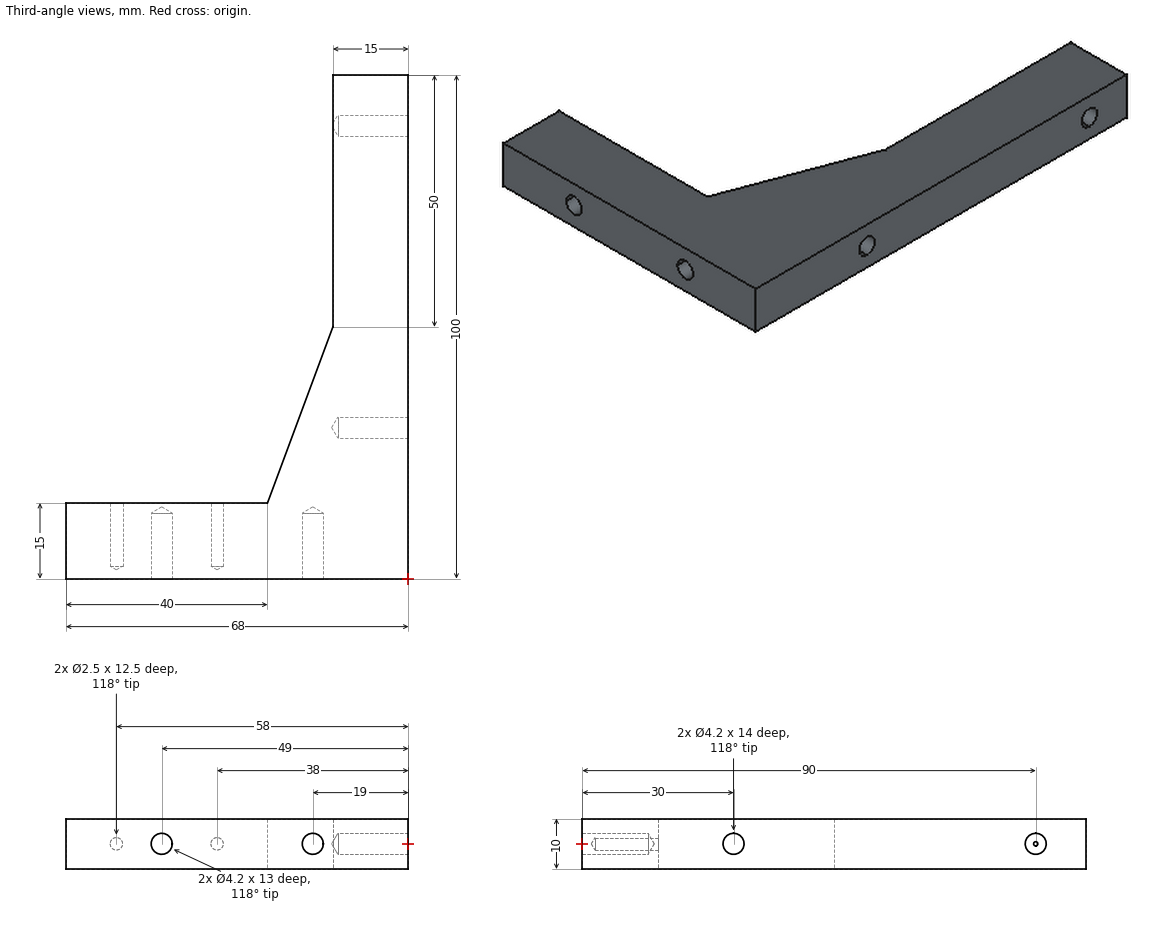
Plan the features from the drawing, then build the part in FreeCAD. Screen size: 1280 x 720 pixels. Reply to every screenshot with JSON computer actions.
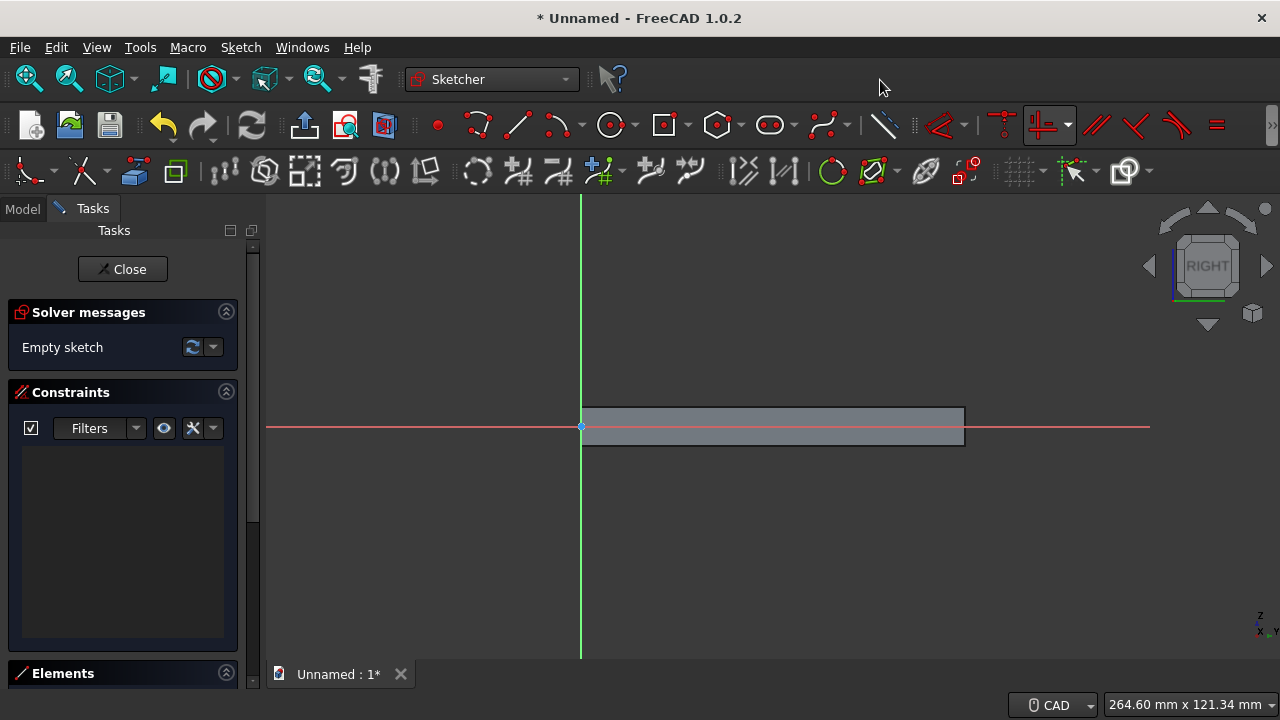
{"action": "scroll", "coordinate": [866, 426], "scroll_direction": "up", "scroll_amount": 2}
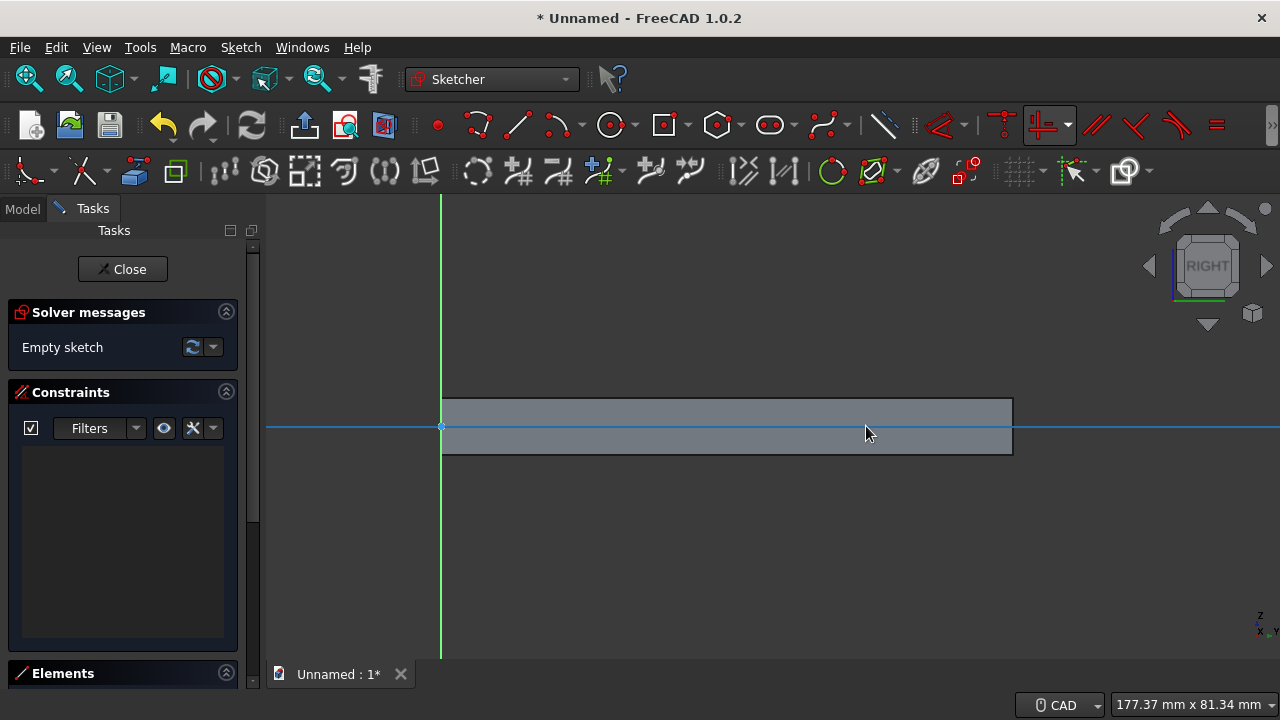
{"action": "key", "text": "g c"}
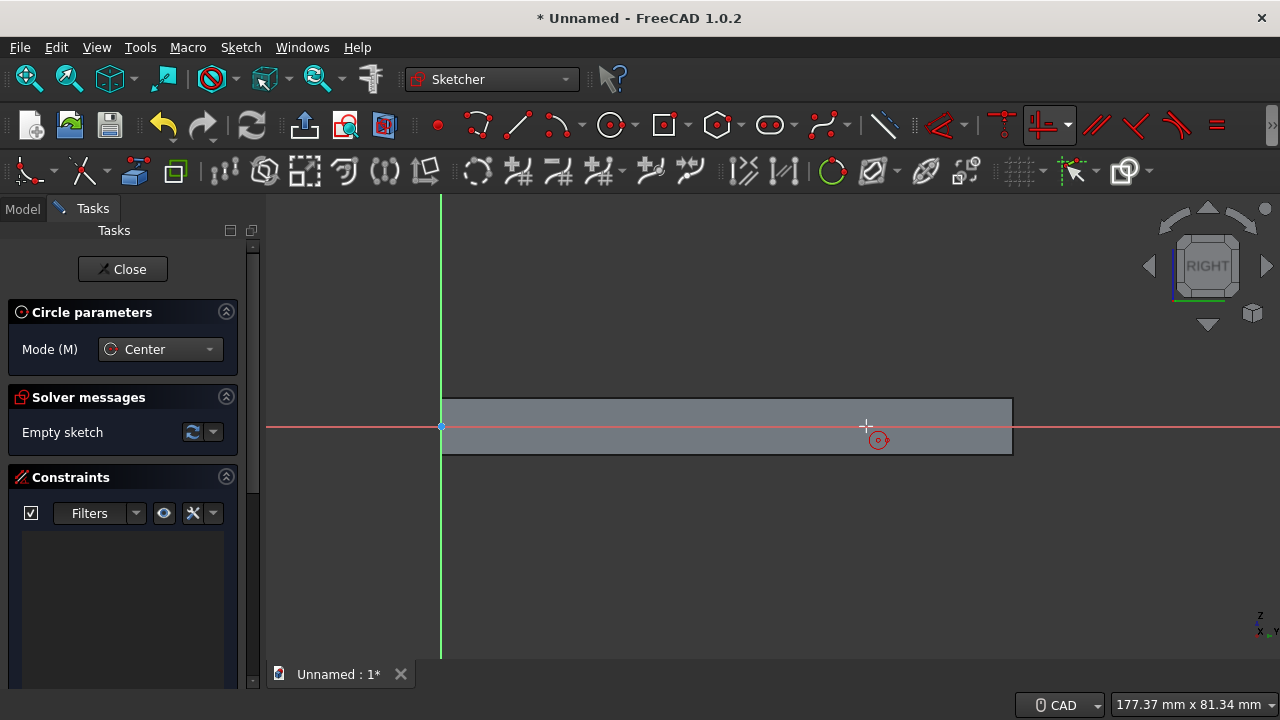
{"action": "scroll", "coordinate": [613, 426], "scroll_direction": "up", "scroll_amount": 4}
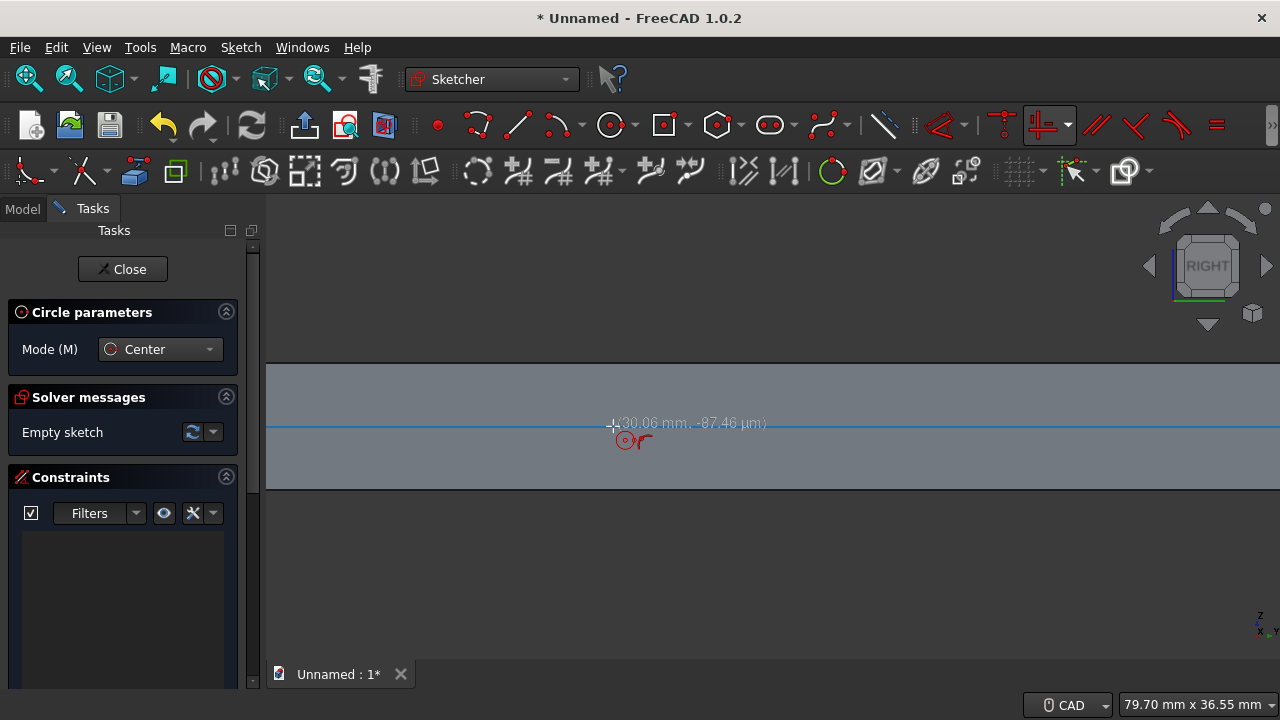
{"action": "left_click", "coordinate": [612, 426]}
{"action": "mouse_move", "coordinate": [631, 408]}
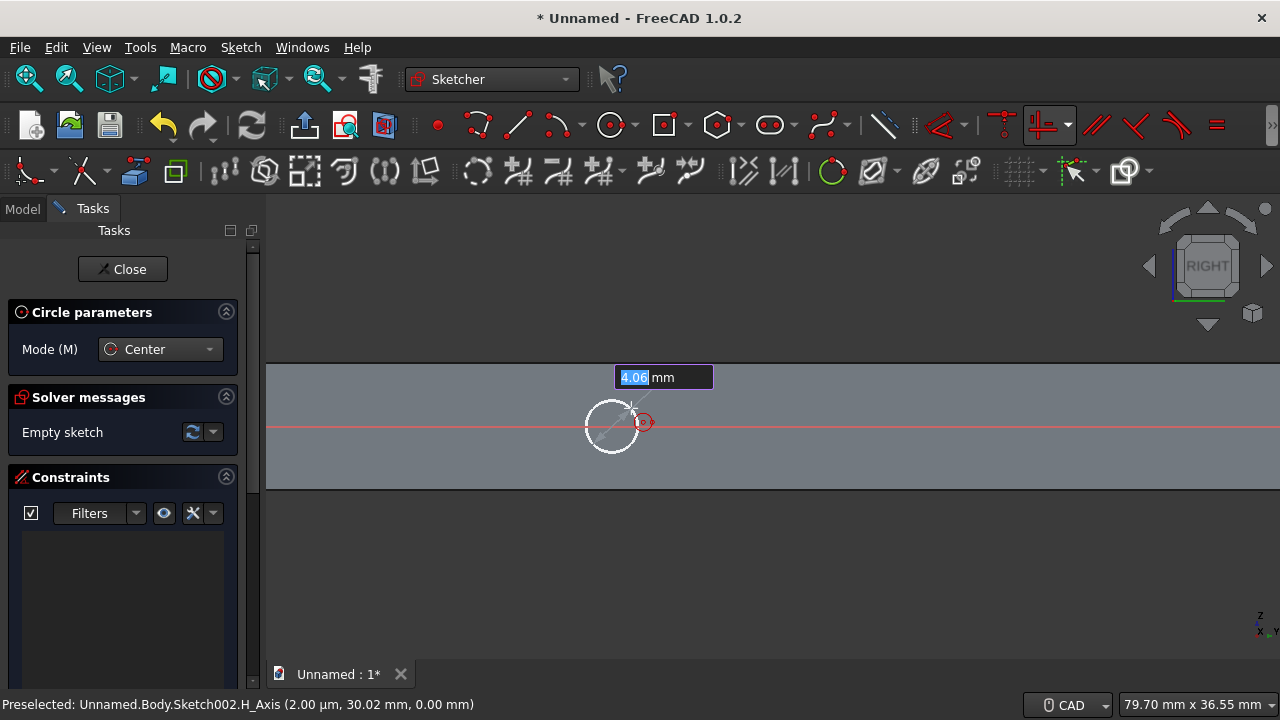
{"action": "type", "text": "4.2"}
{"action": "key", "text": "Return"}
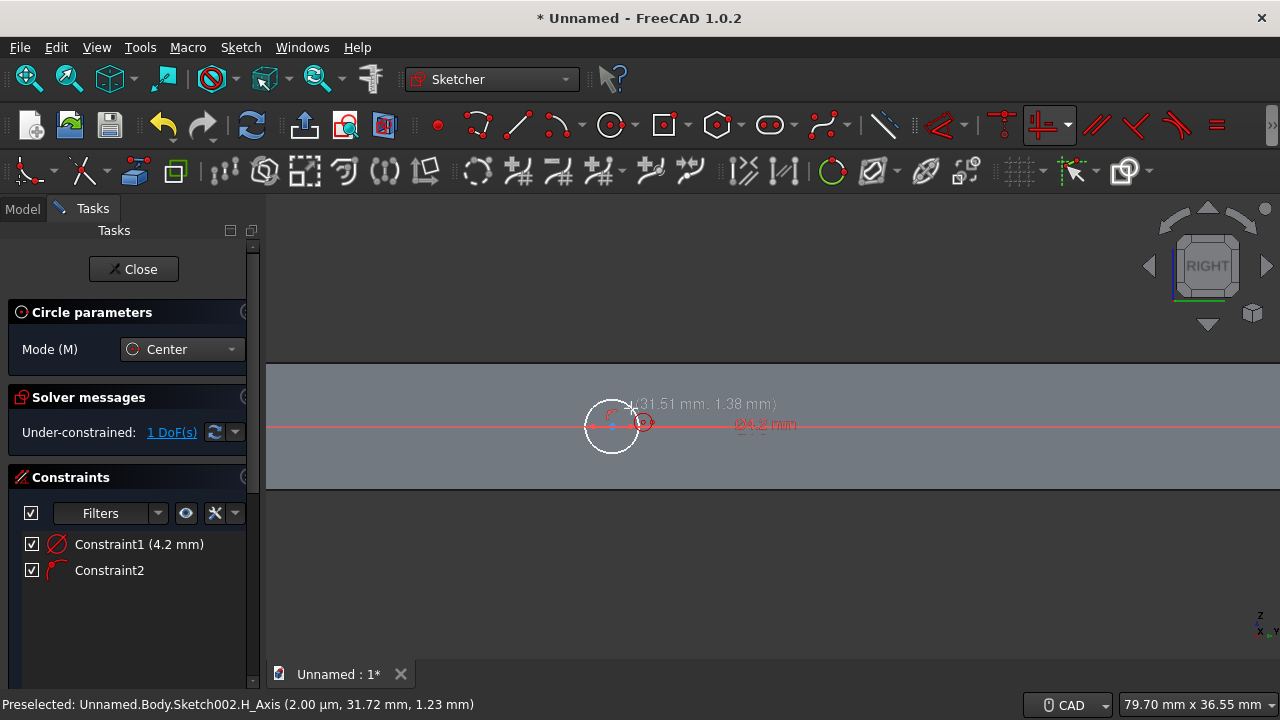
{"action": "scroll", "coordinate": [614, 426], "scroll_direction": "down", "scroll_amount": 4}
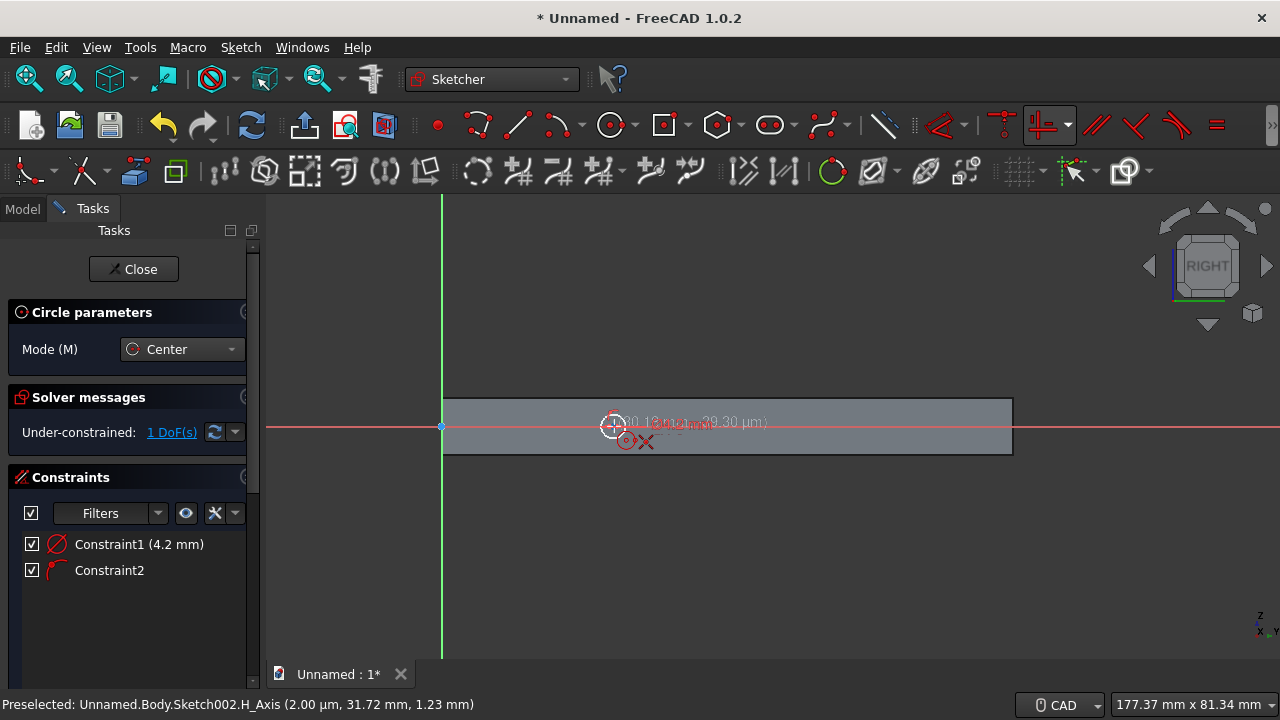
{"action": "scroll", "coordinate": [956, 426], "scroll_direction": "up", "scroll_amount": 4}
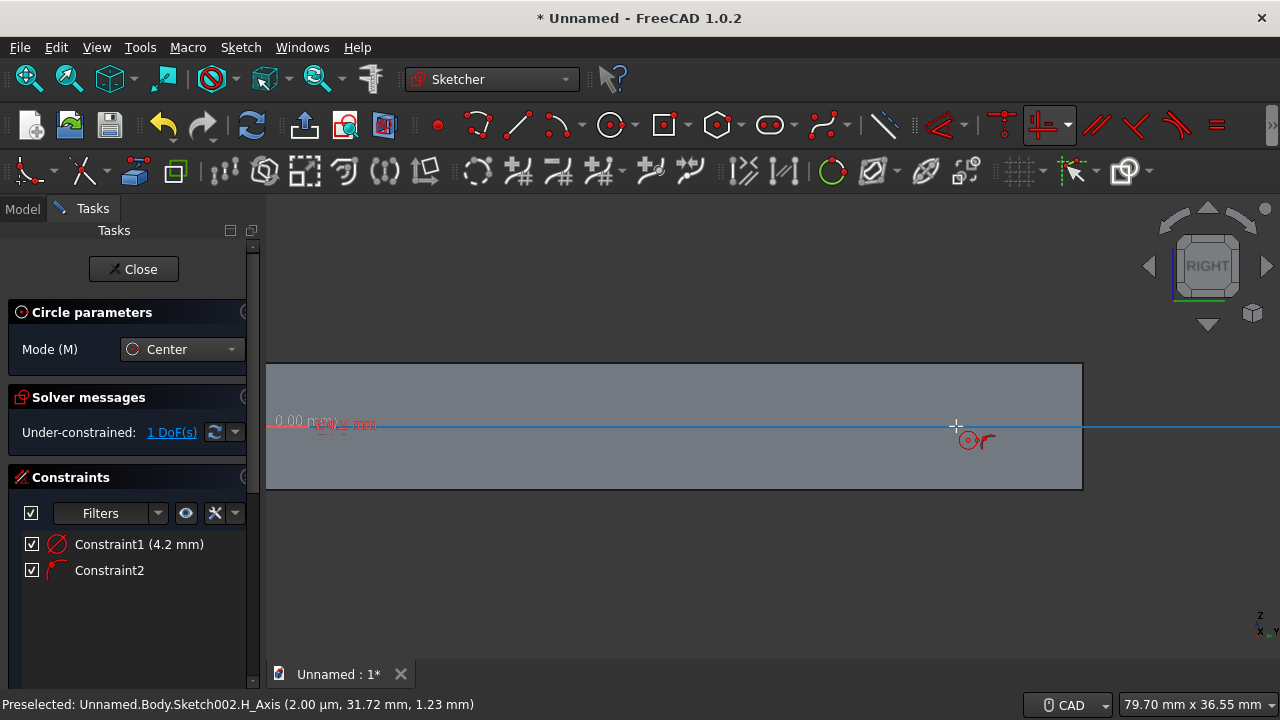
{"action": "left_click", "coordinate": [956, 426]}
{"action": "mouse_move", "coordinate": [974, 408]}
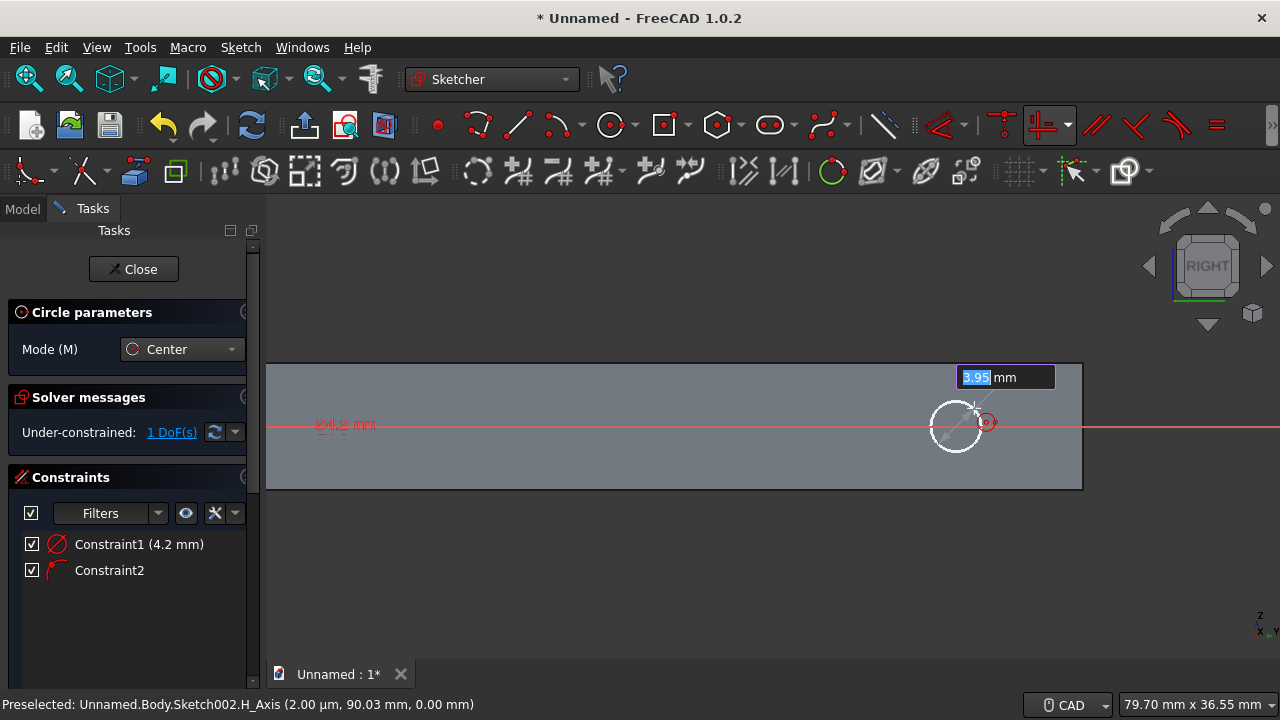
{"action": "type", "text": "4.2"}
{"action": "key", "text": "Return"}
{"action": "key", "text": "Escape"}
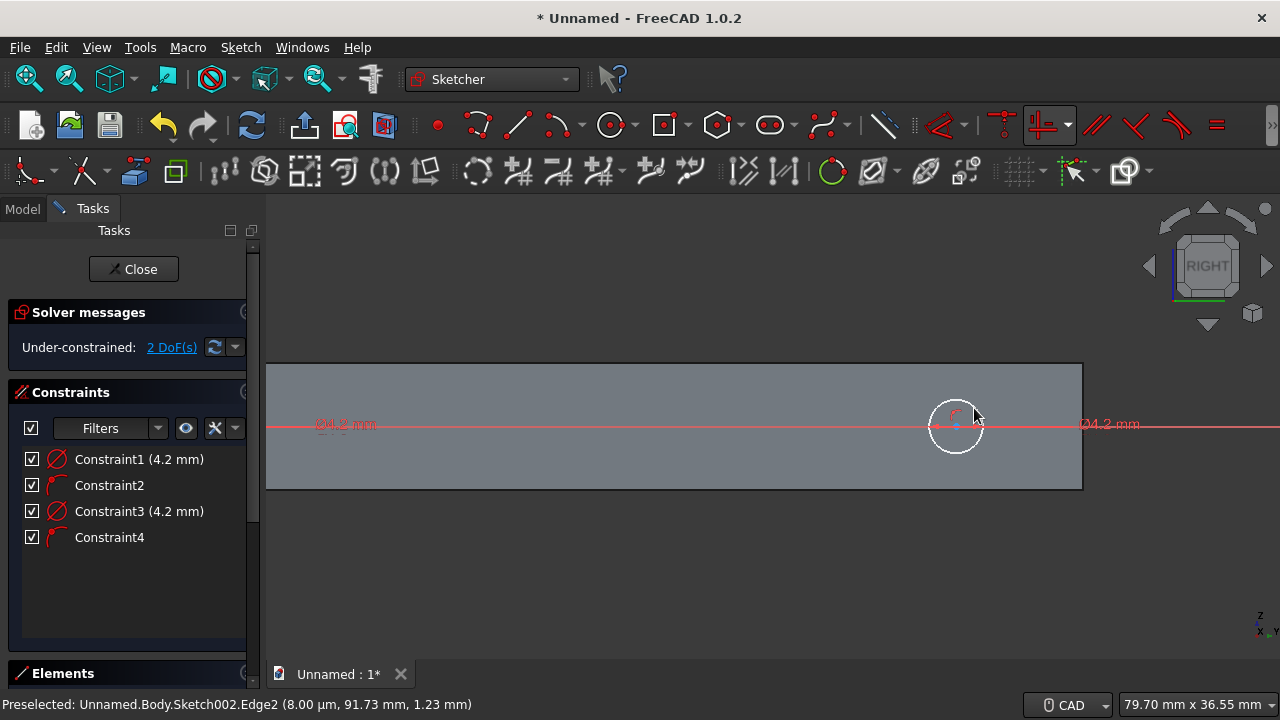
{"action": "key", "text": "d"}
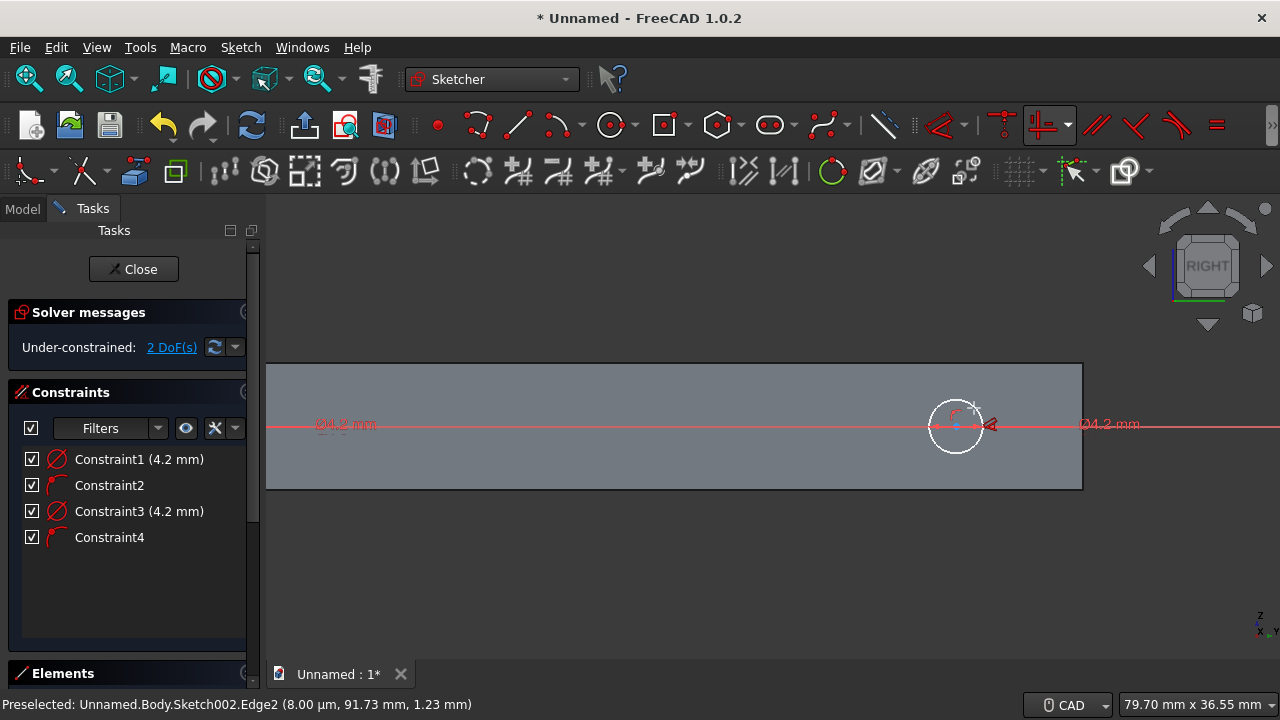
{"action": "scroll", "coordinate": [956, 426], "scroll_direction": "down", "scroll_amount": 4}